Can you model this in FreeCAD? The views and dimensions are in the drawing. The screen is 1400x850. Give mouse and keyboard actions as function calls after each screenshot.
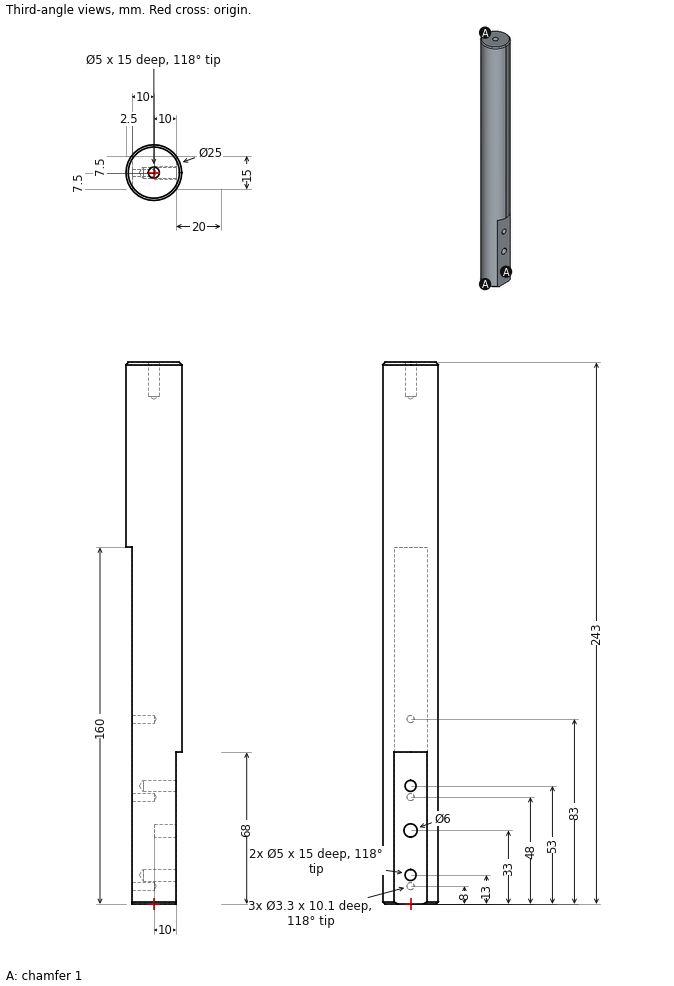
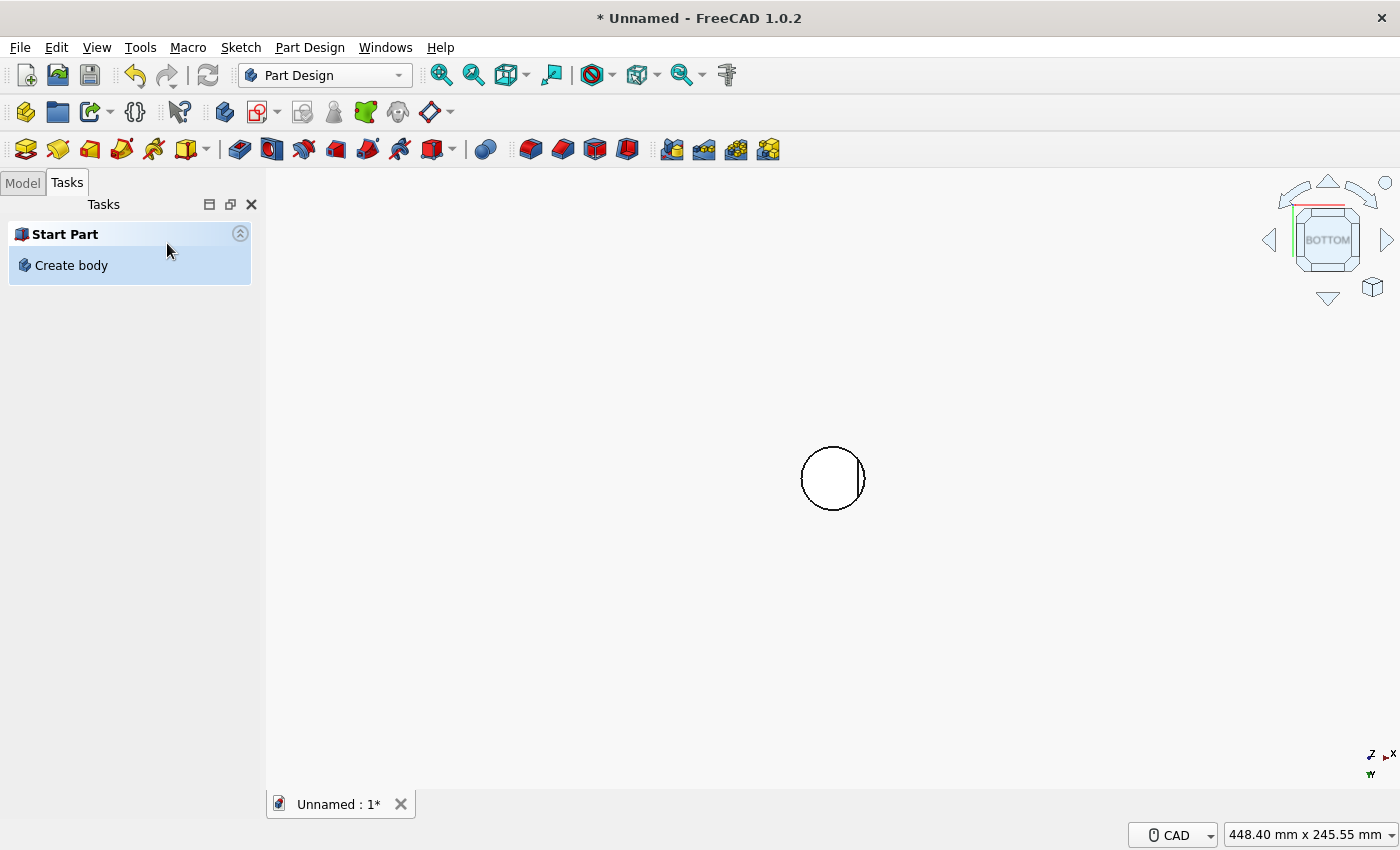
click(830, 477)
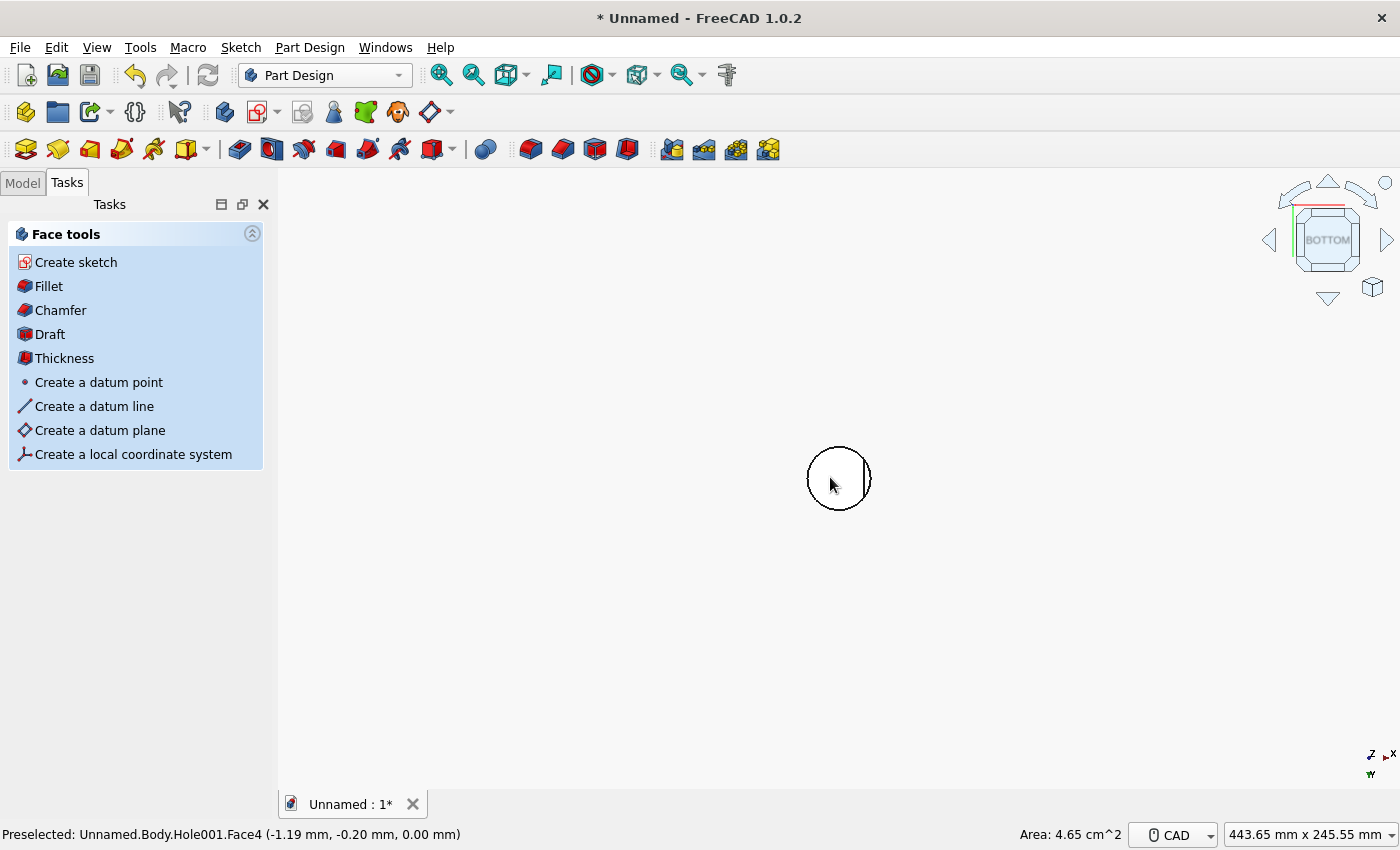
click(258, 112)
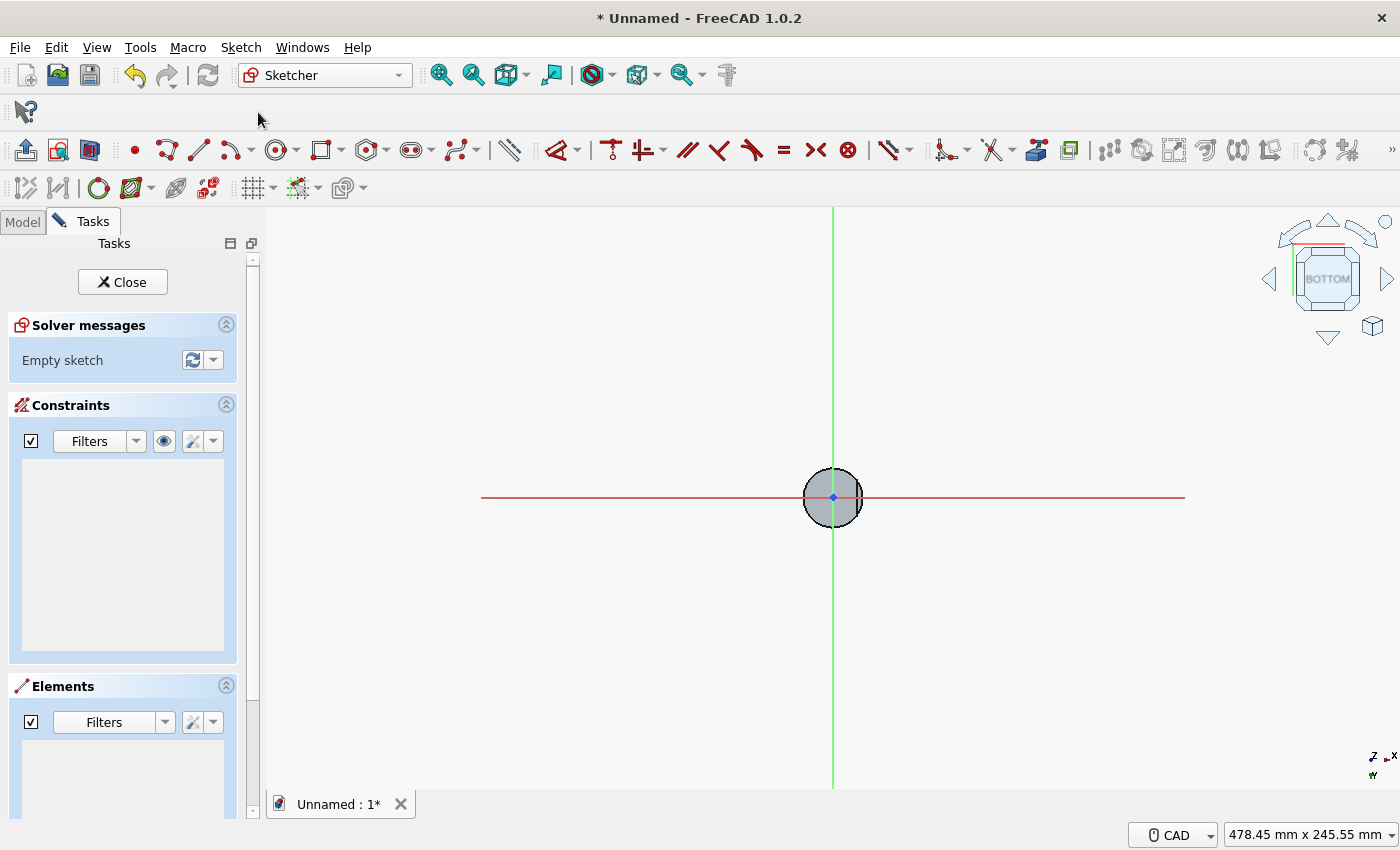
scroll(824, 498, up, 12)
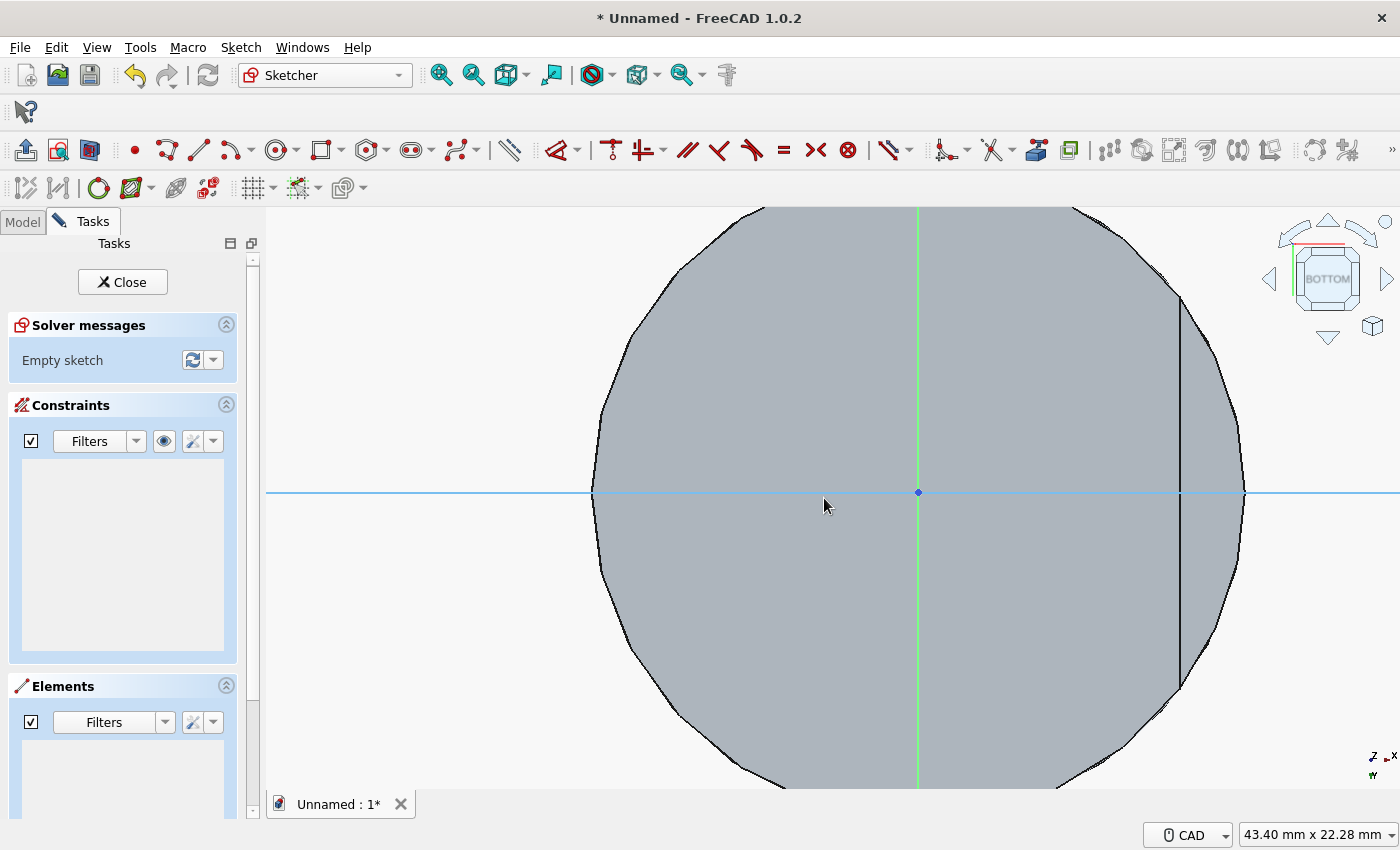
key(g)
key(r)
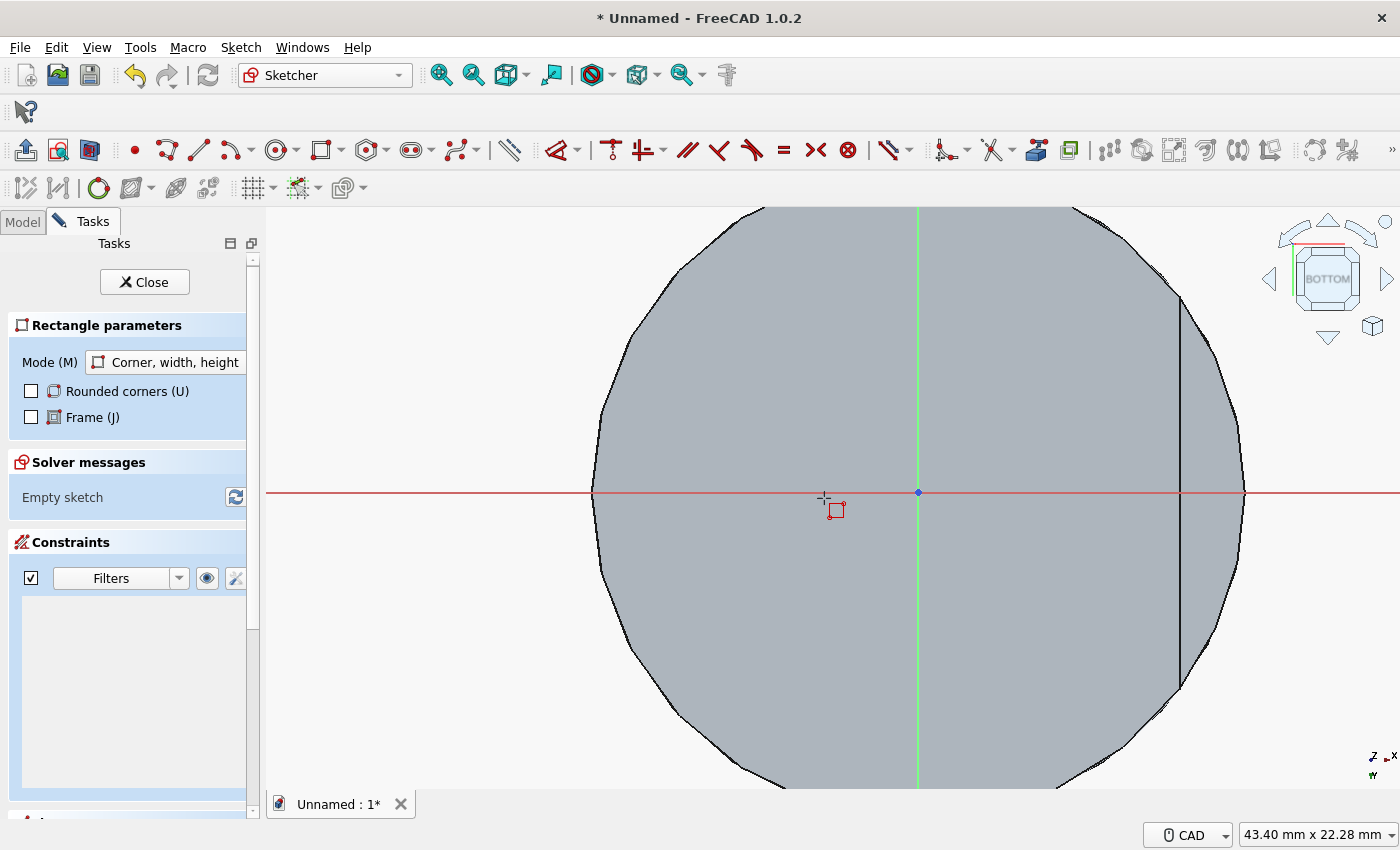
click(592, 297)
click(657, 689)
key(Escape)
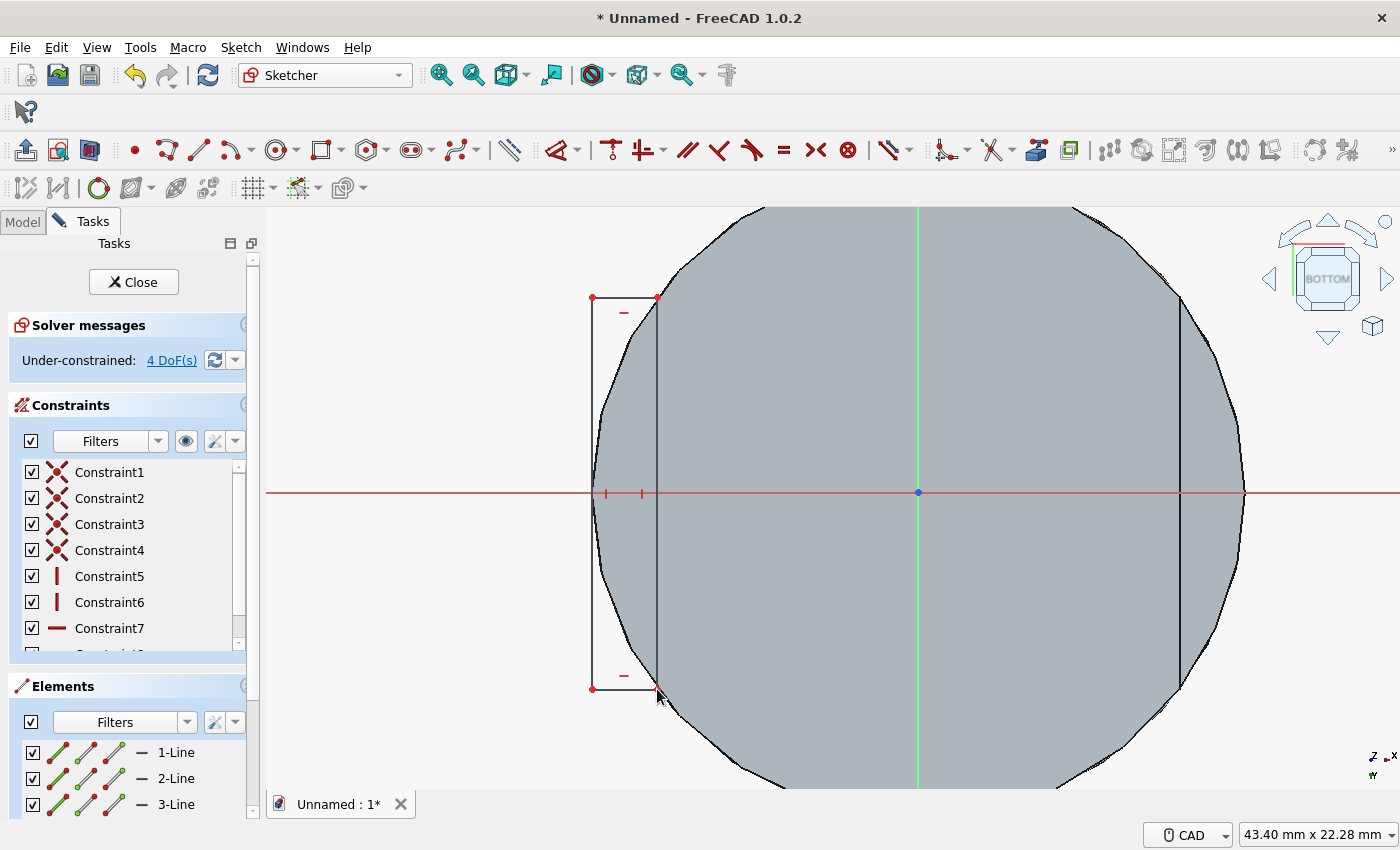
click(556, 150)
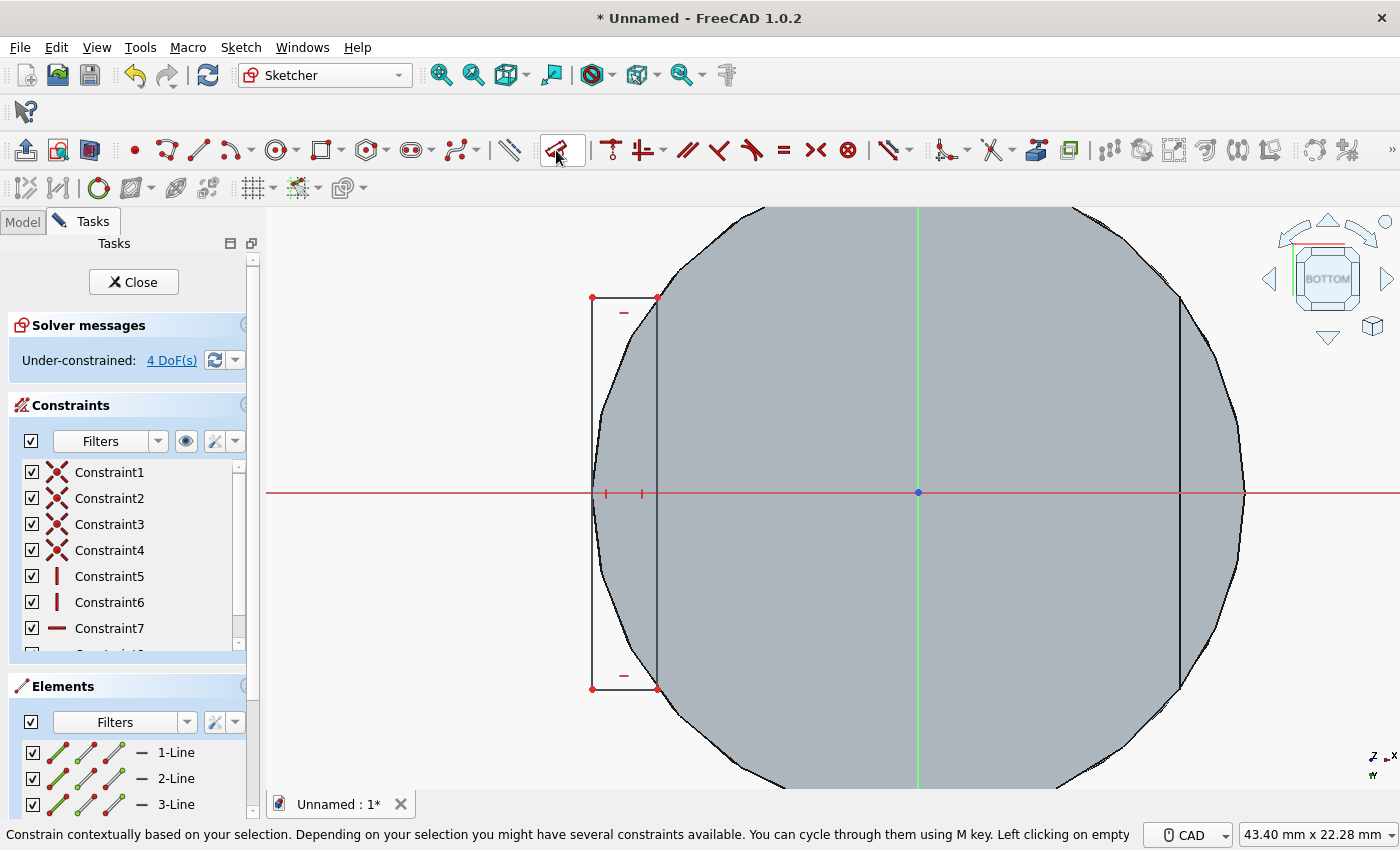
click(592, 416)
click(558, 404)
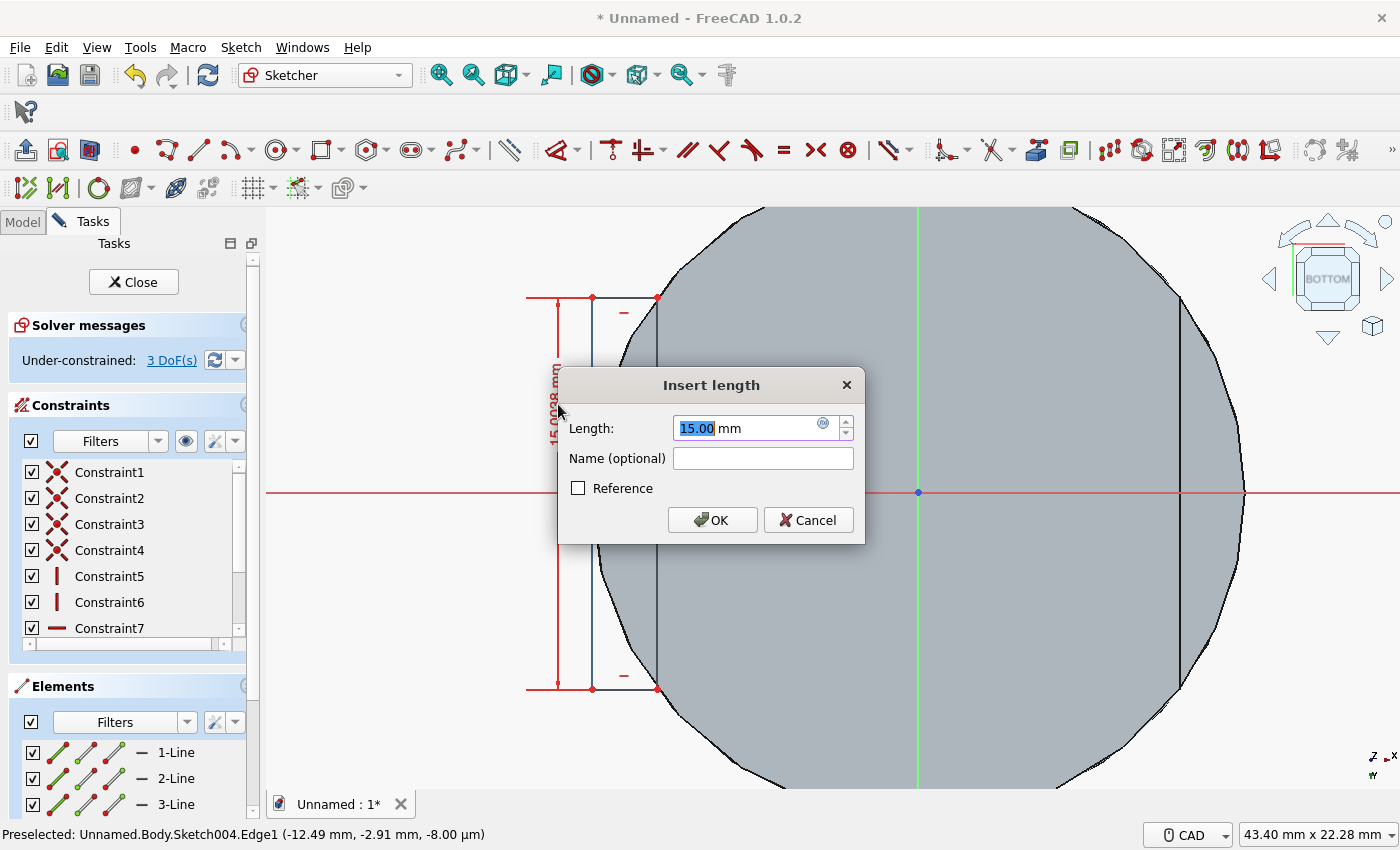
text(15)
key(Return)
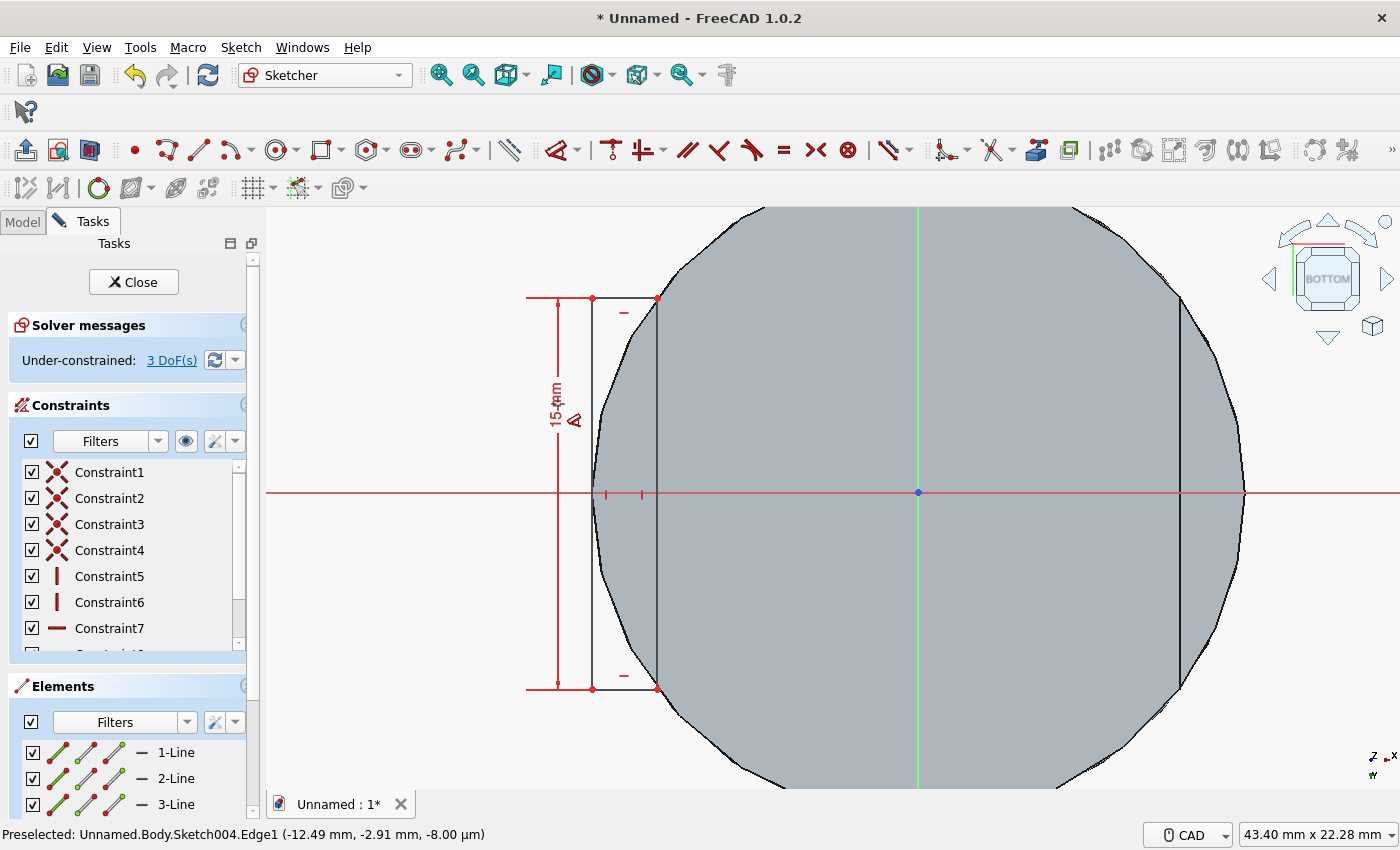
click(611, 690)
click(624, 724)